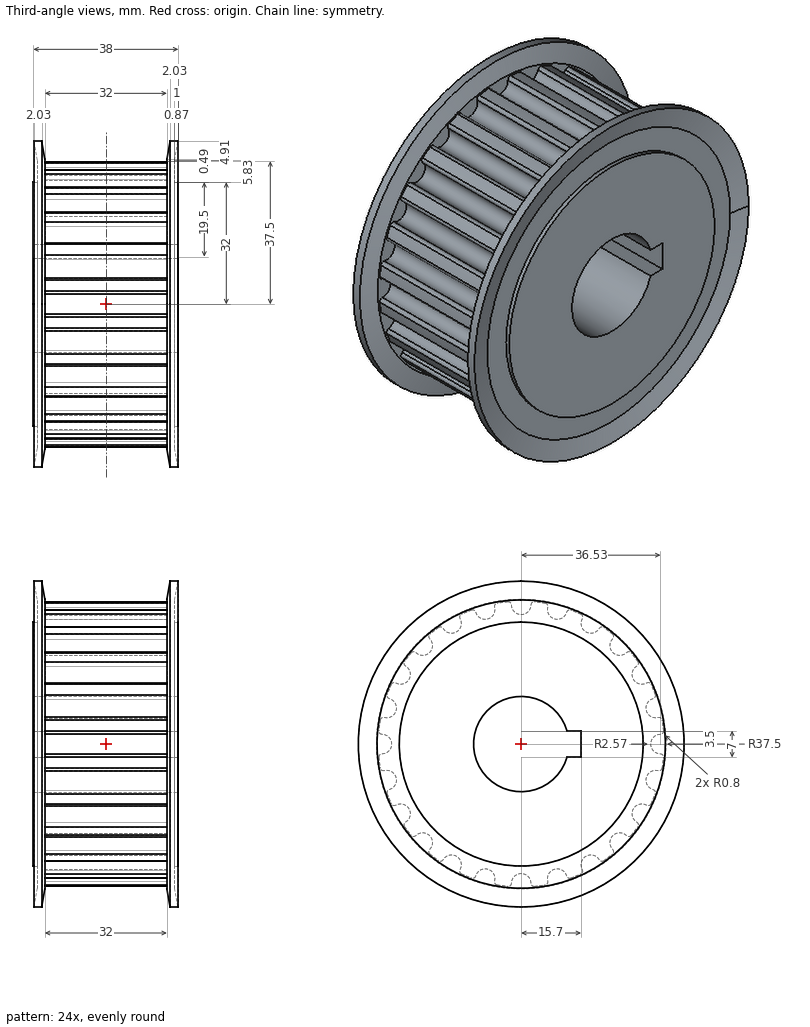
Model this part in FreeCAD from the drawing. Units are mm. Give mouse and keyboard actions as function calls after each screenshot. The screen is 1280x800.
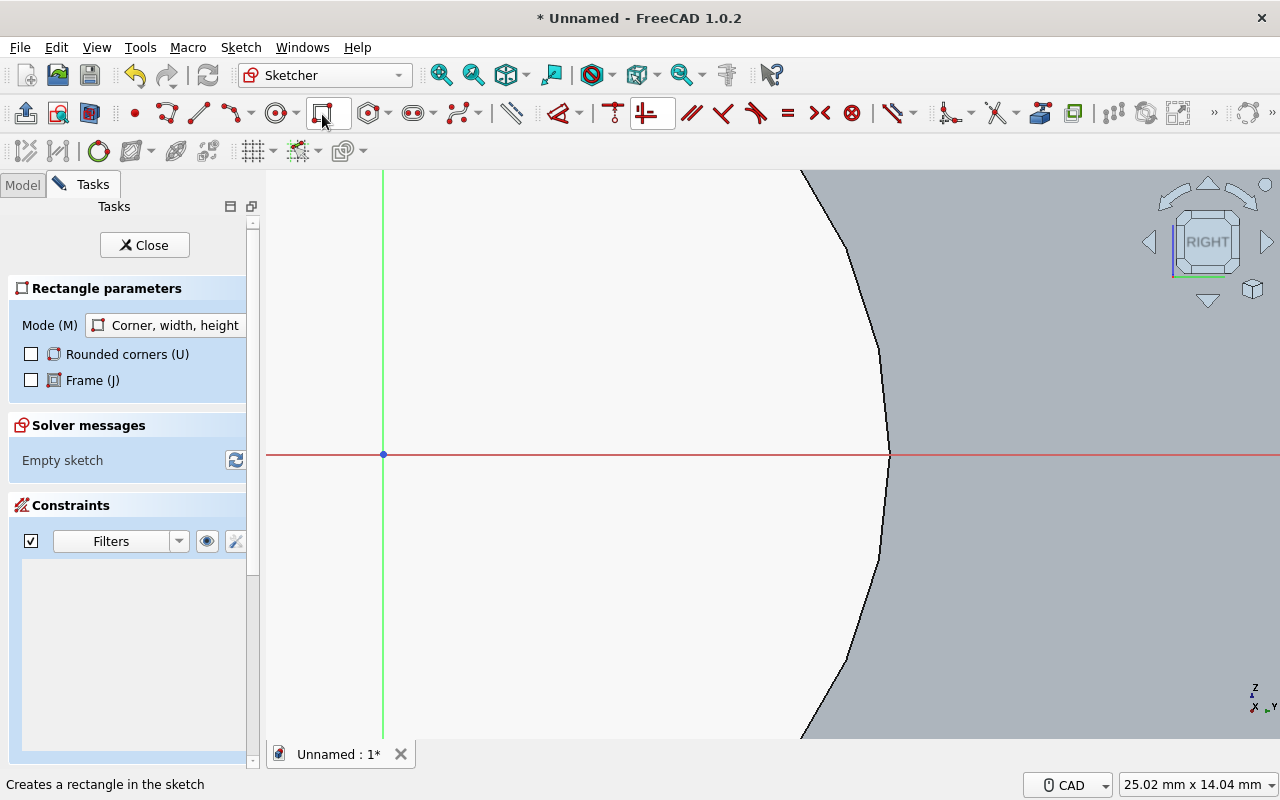
click(383, 313)
click(1020, 596)
key(Escape)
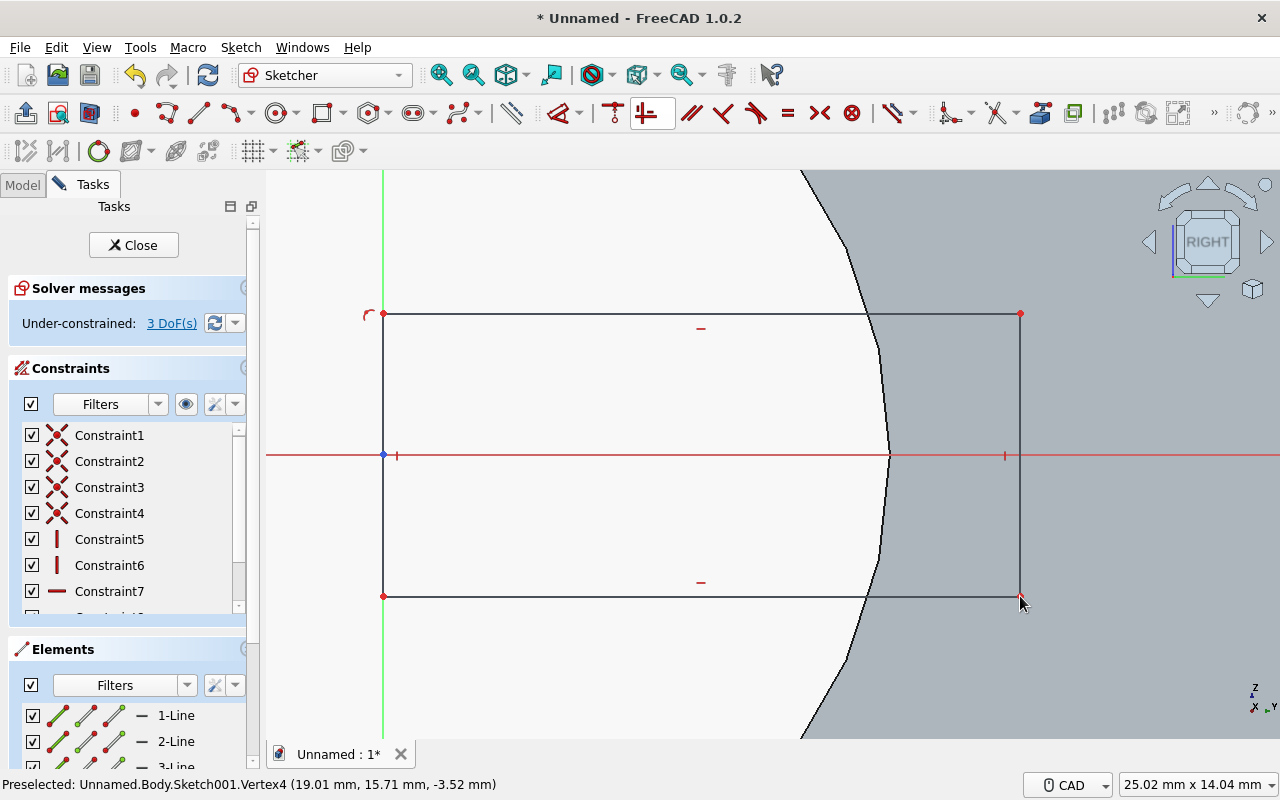
click(558, 114)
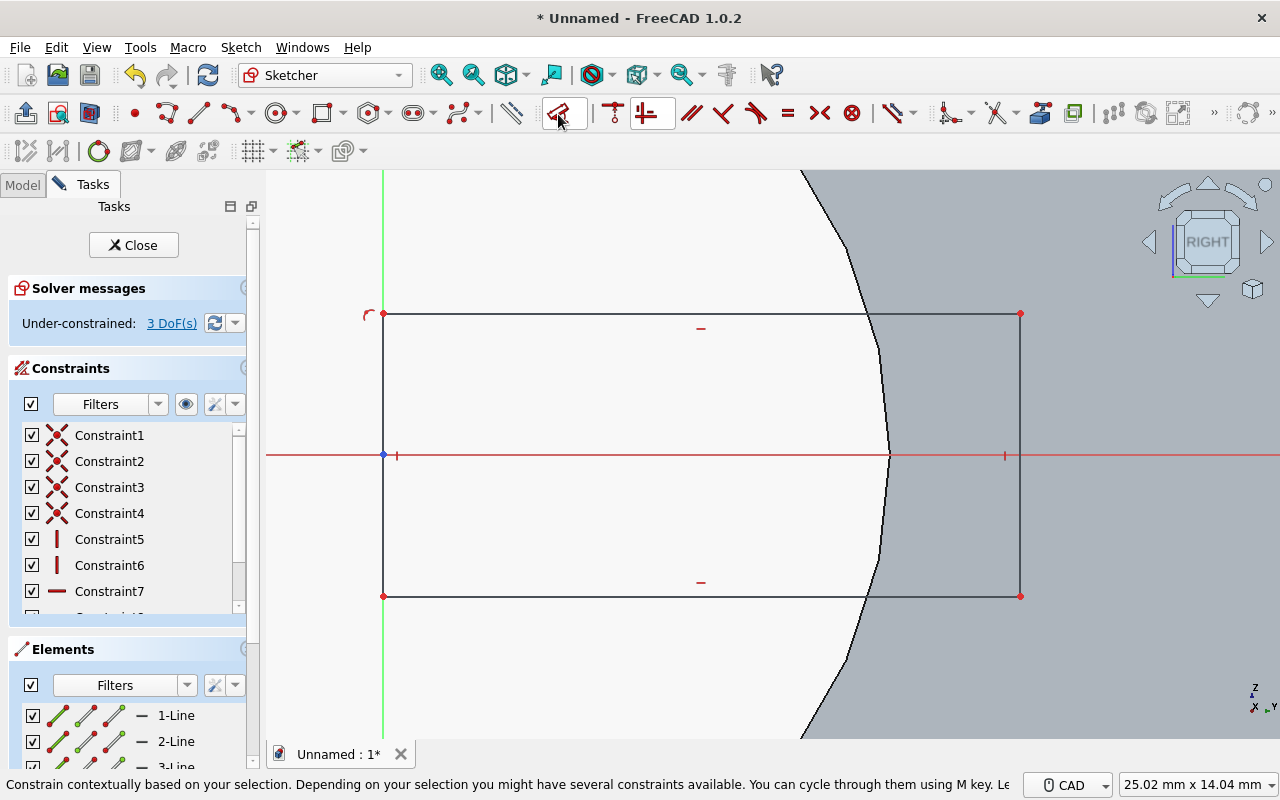
click(383, 399)
click(349, 390)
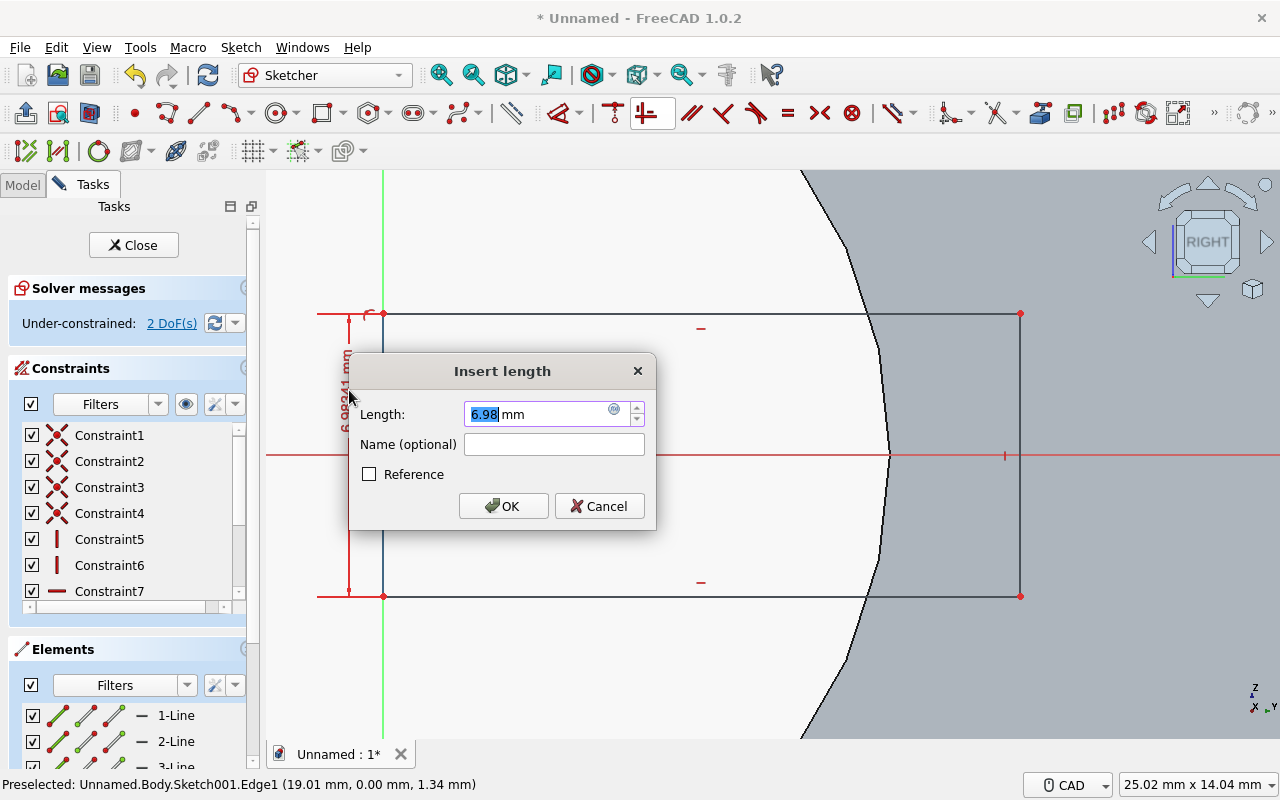
text(7)
key(Return)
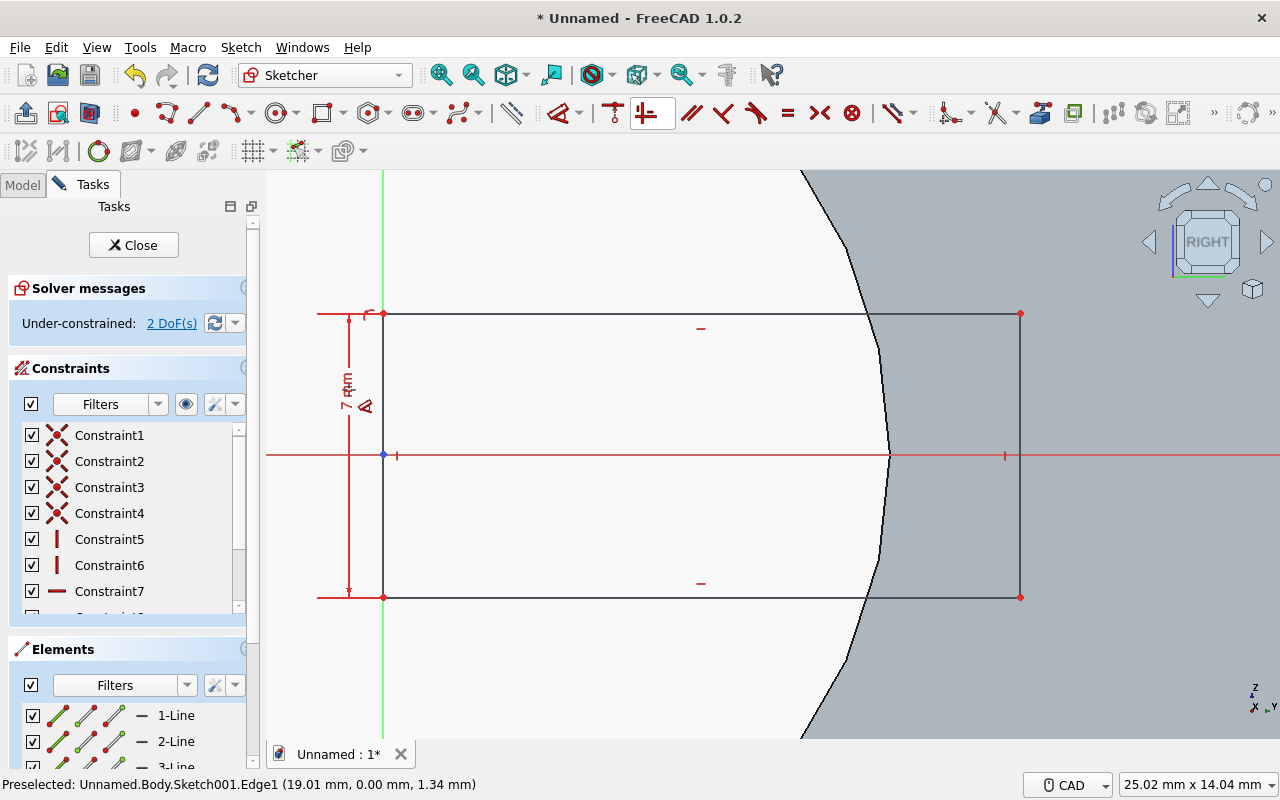
click(574, 598)
click(702, 632)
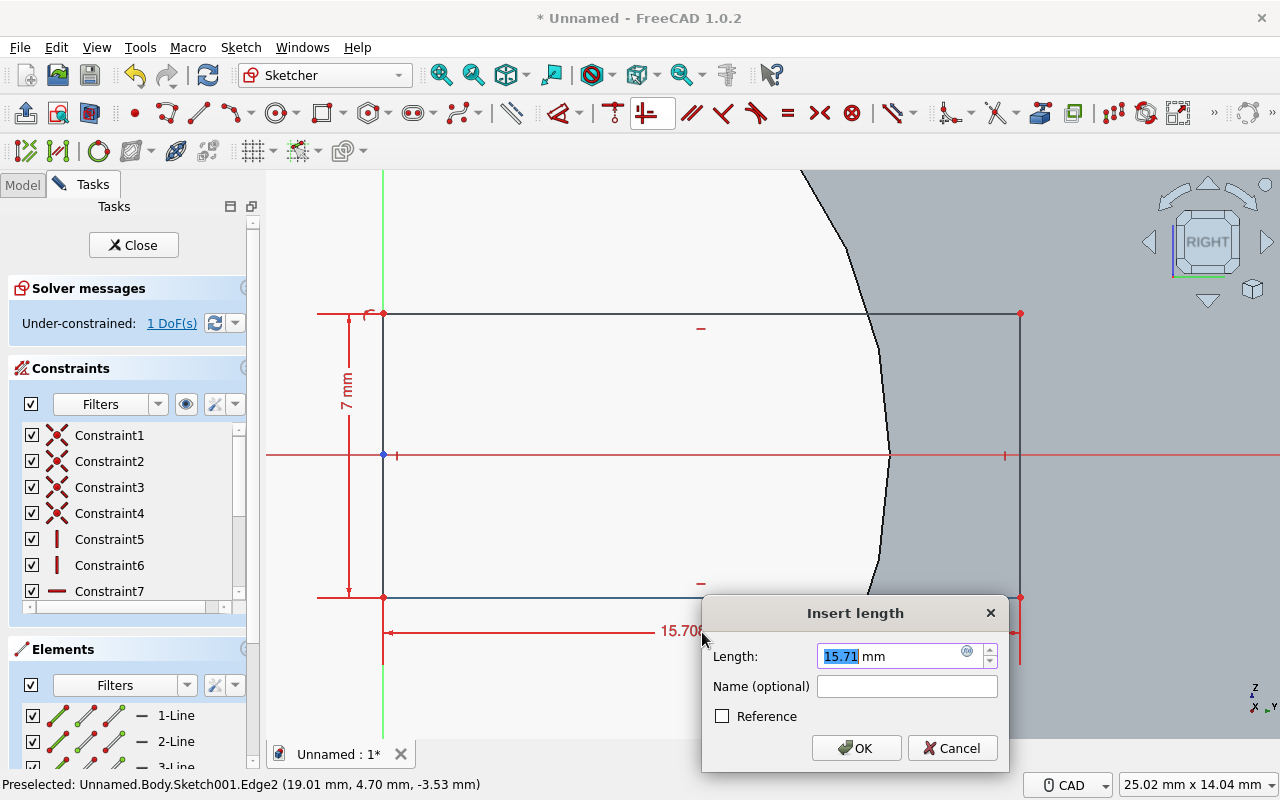
text(15.7)
key(Return)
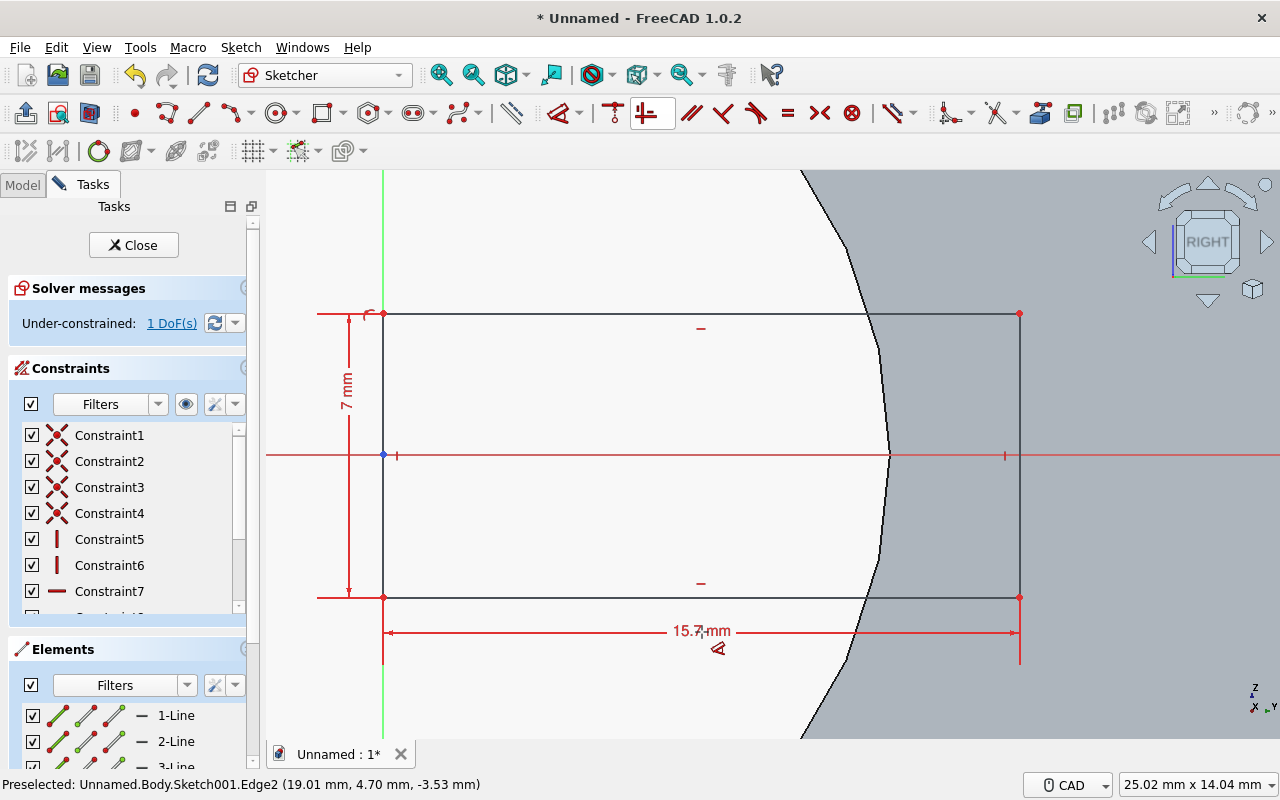
click(383, 314)
click(349, 352)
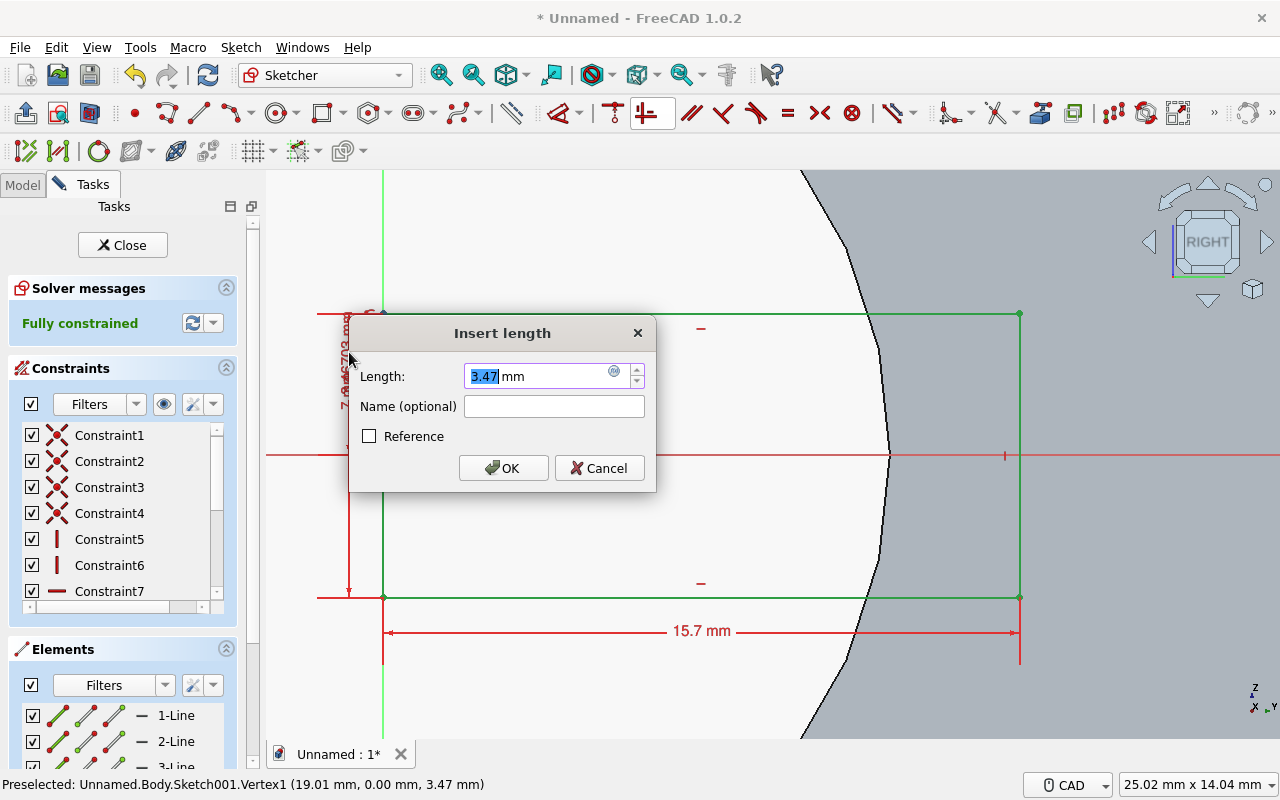
text(3.5)
key(Return)
key(Escape)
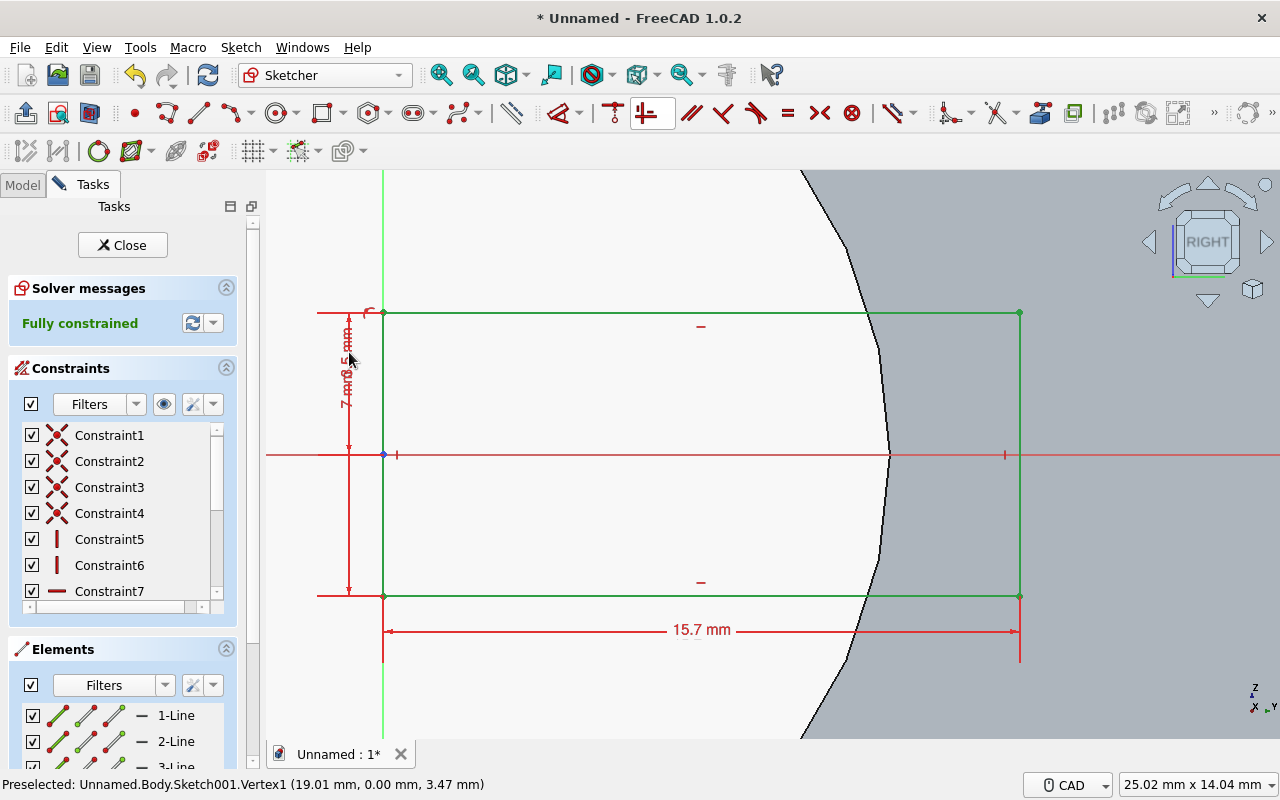
click(123, 245)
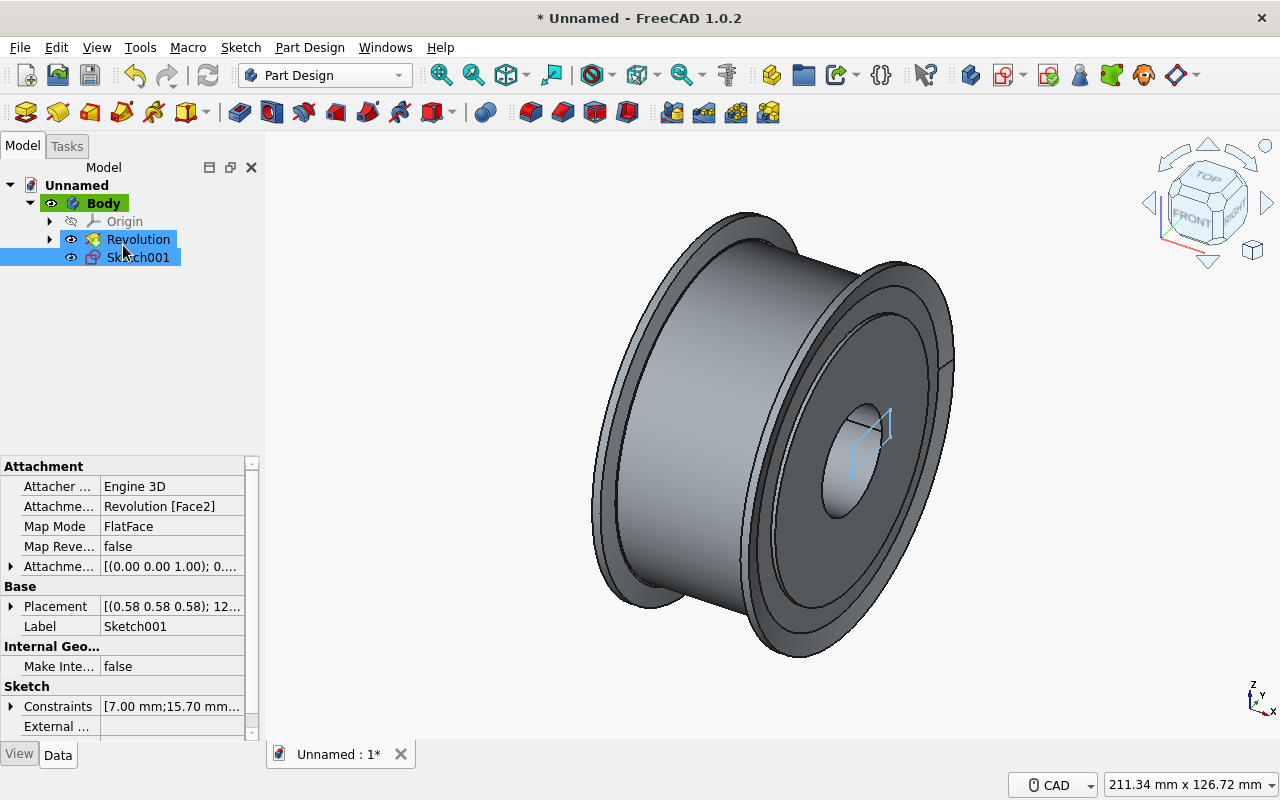
click(240, 112)